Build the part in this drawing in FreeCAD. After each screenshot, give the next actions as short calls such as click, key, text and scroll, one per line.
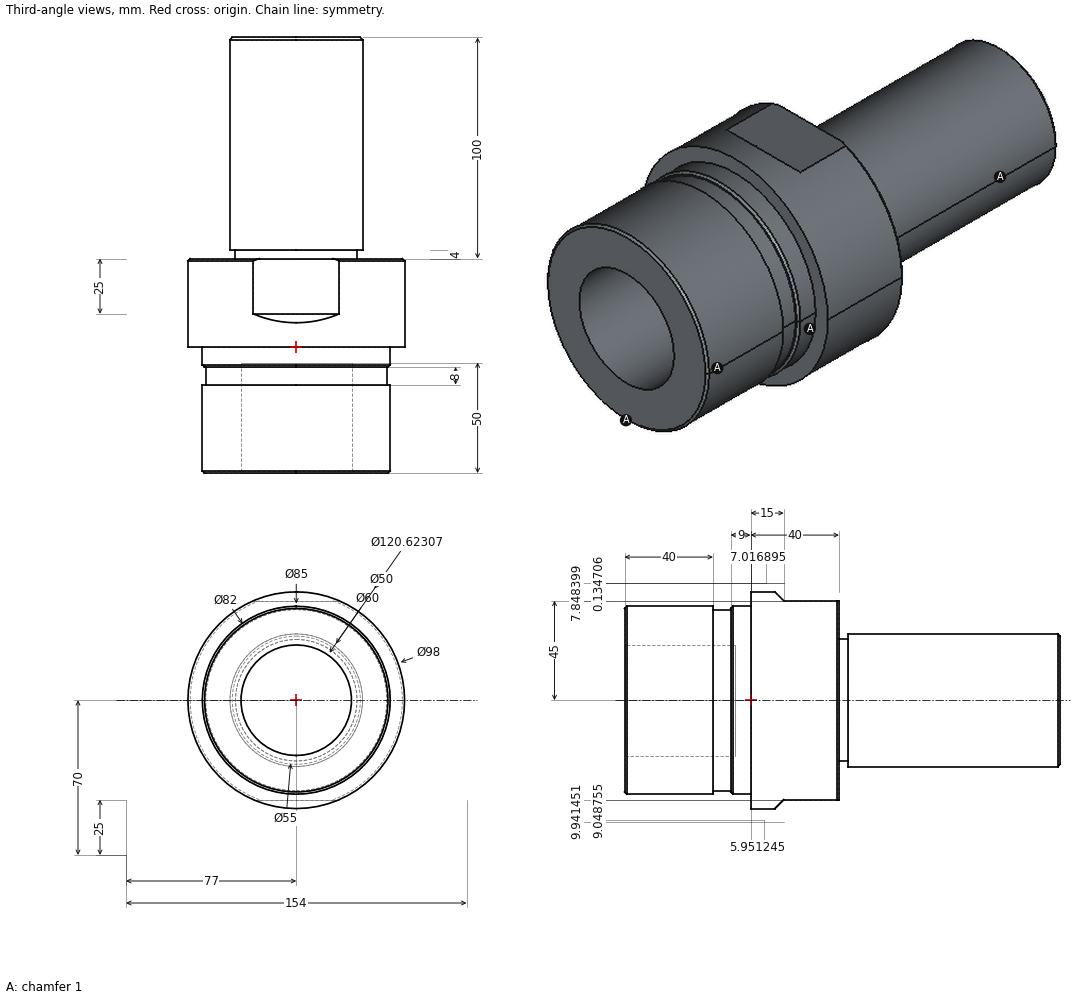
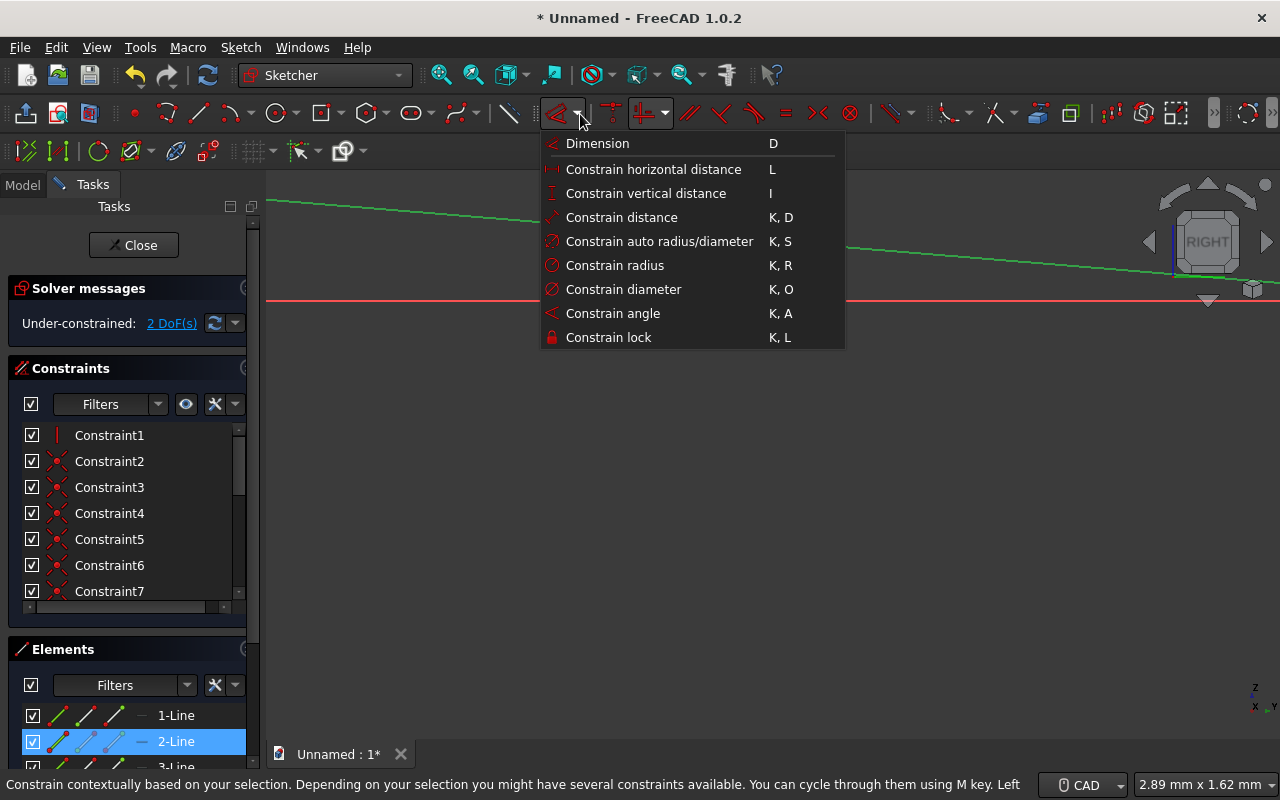
click(693, 193)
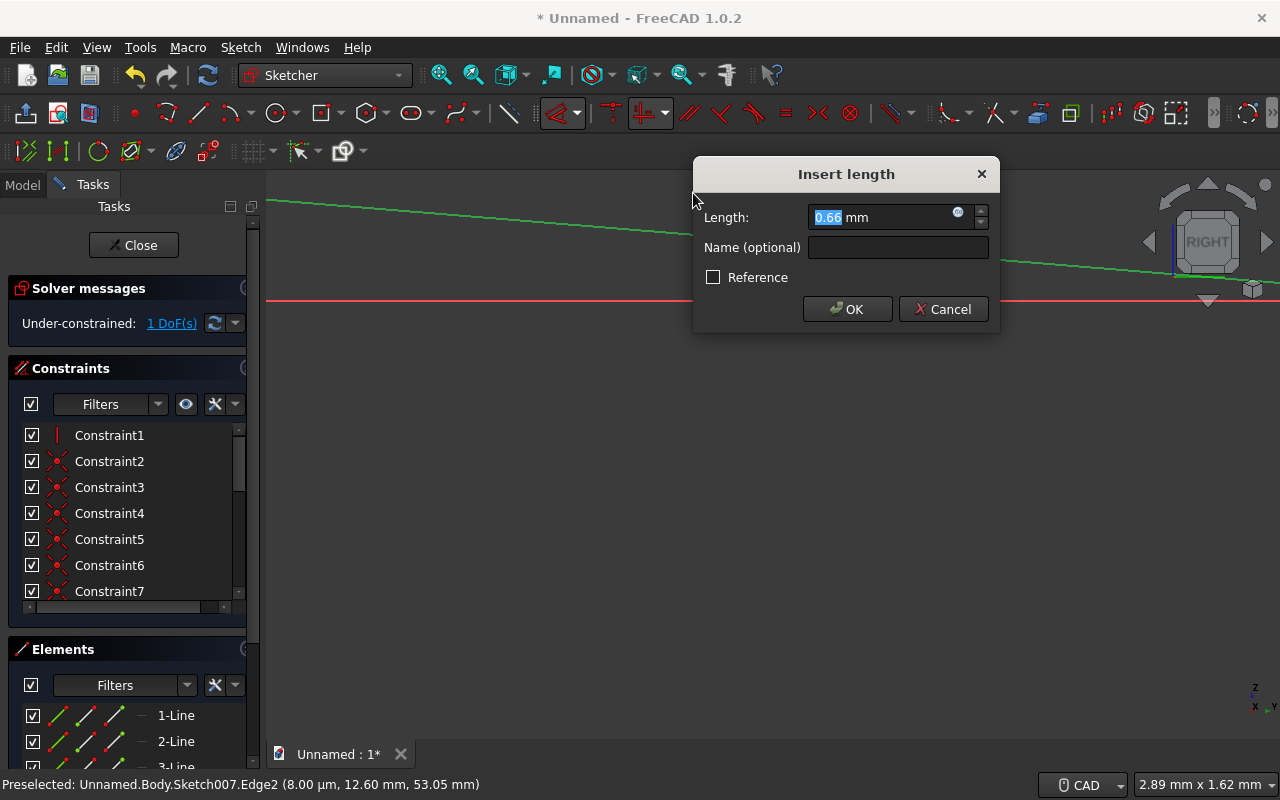
text(0.134706)
key(Return)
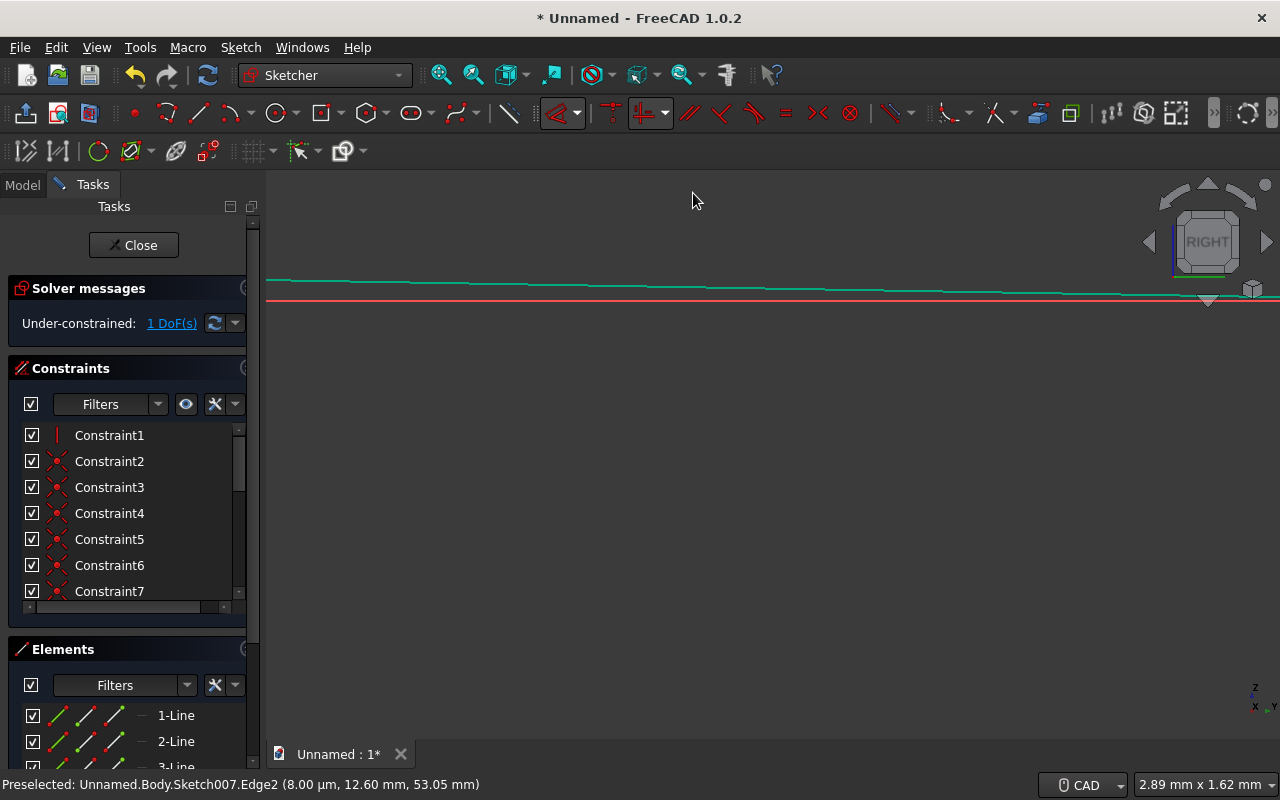
scroll(704, 454, down, 15)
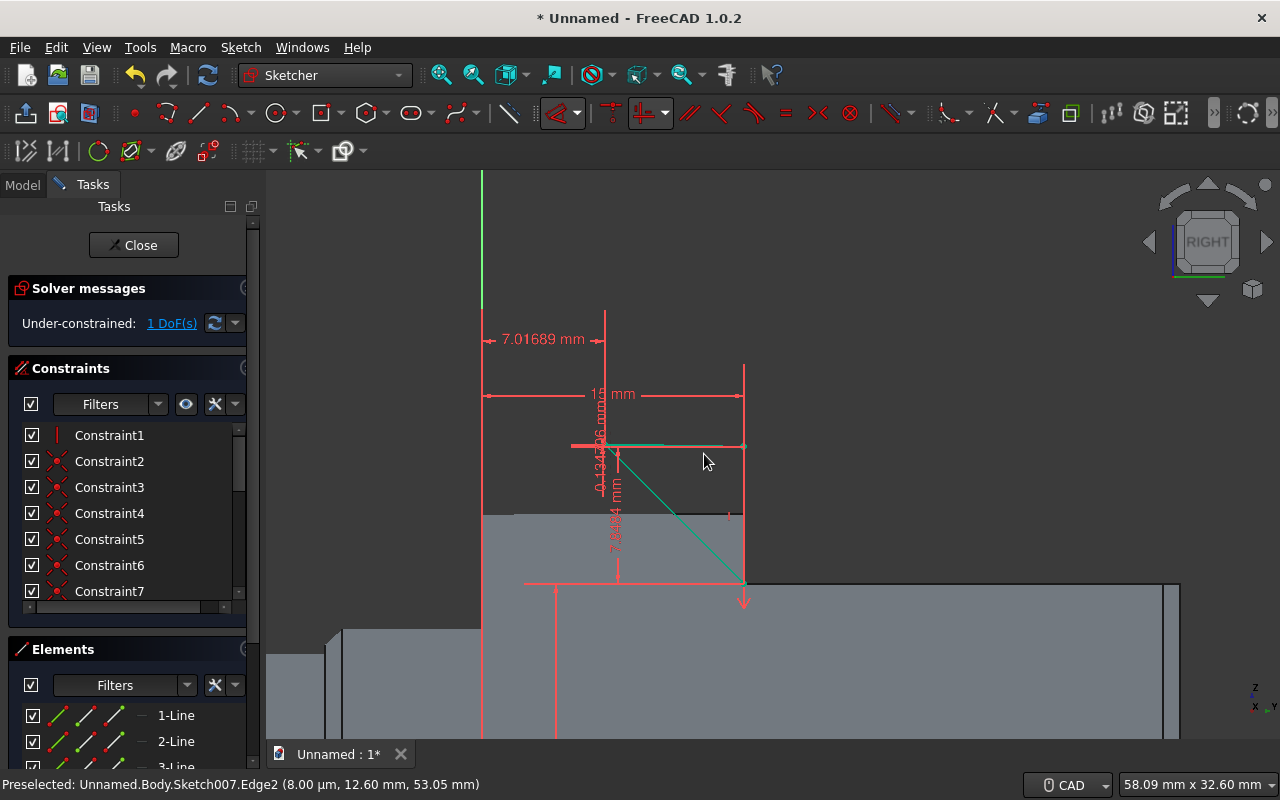
scroll(728, 219, down, 8)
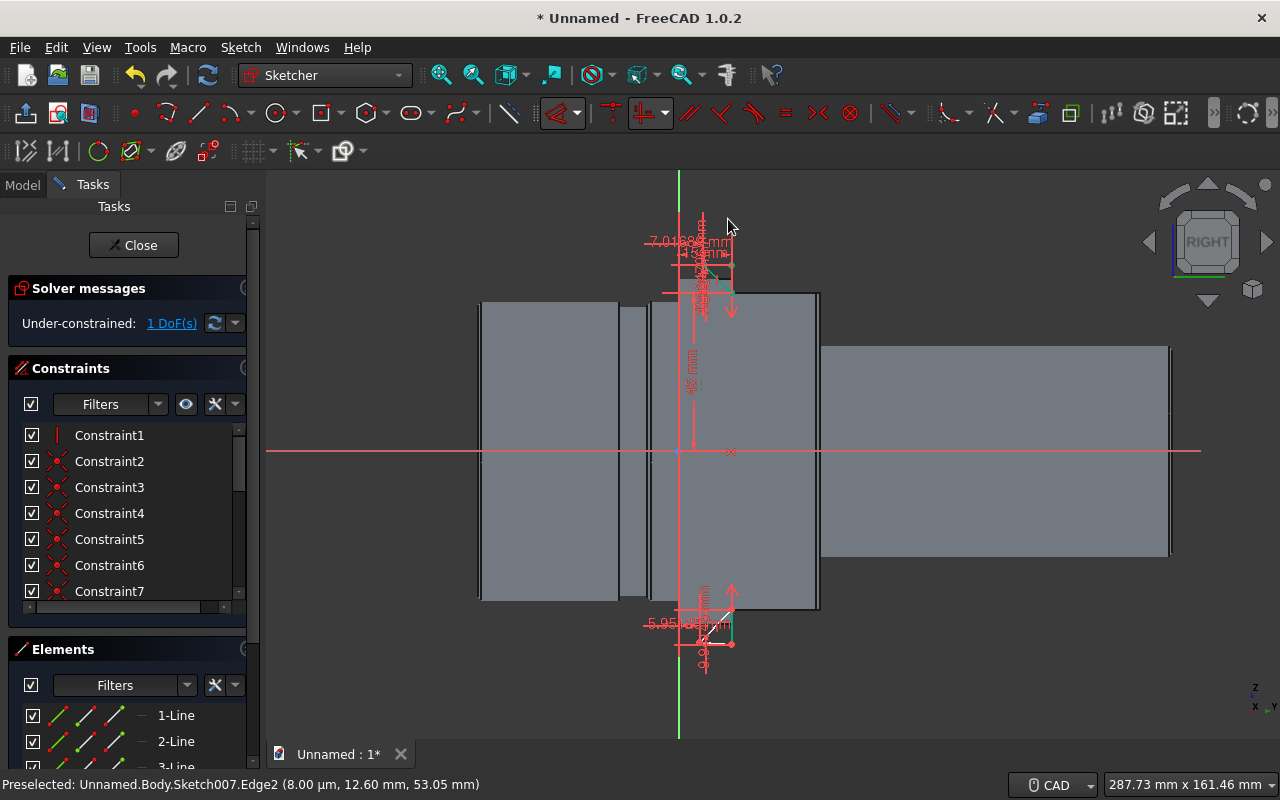
scroll(722, 620, up, 2)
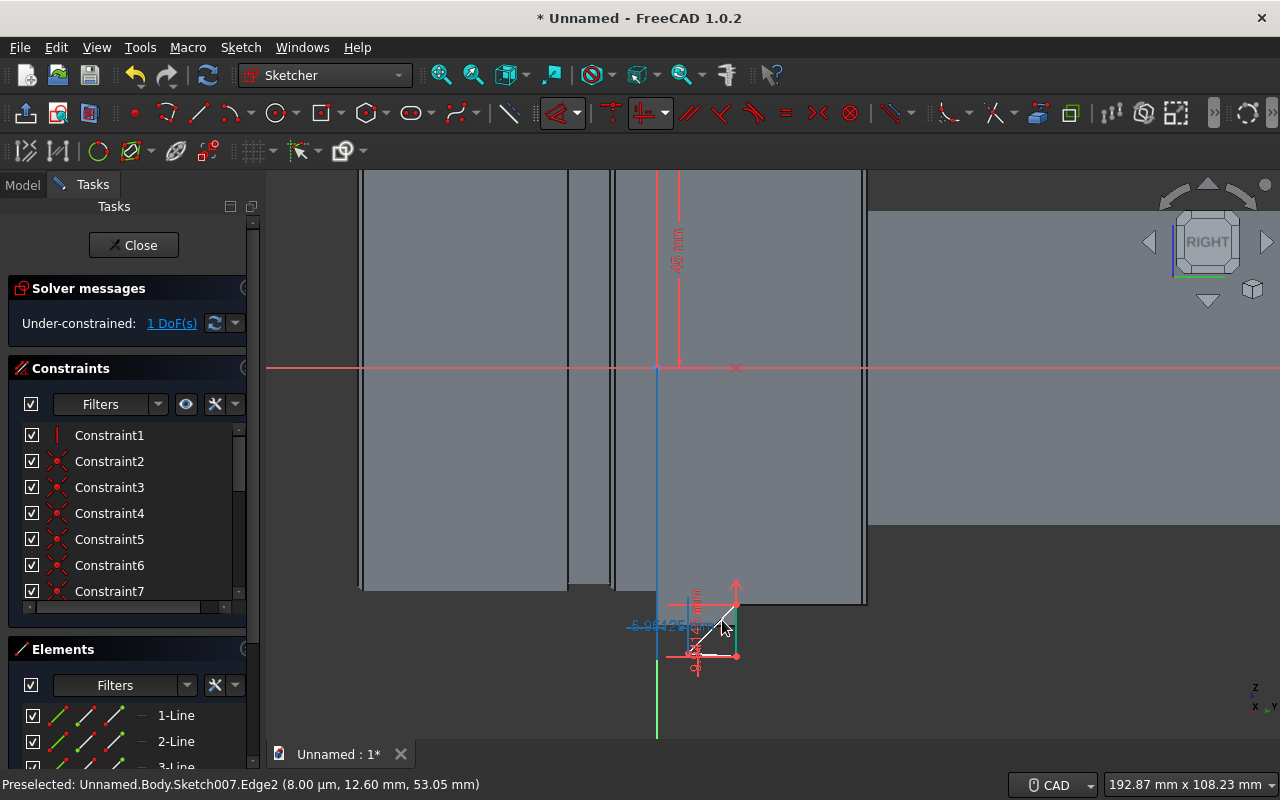
click(722, 619)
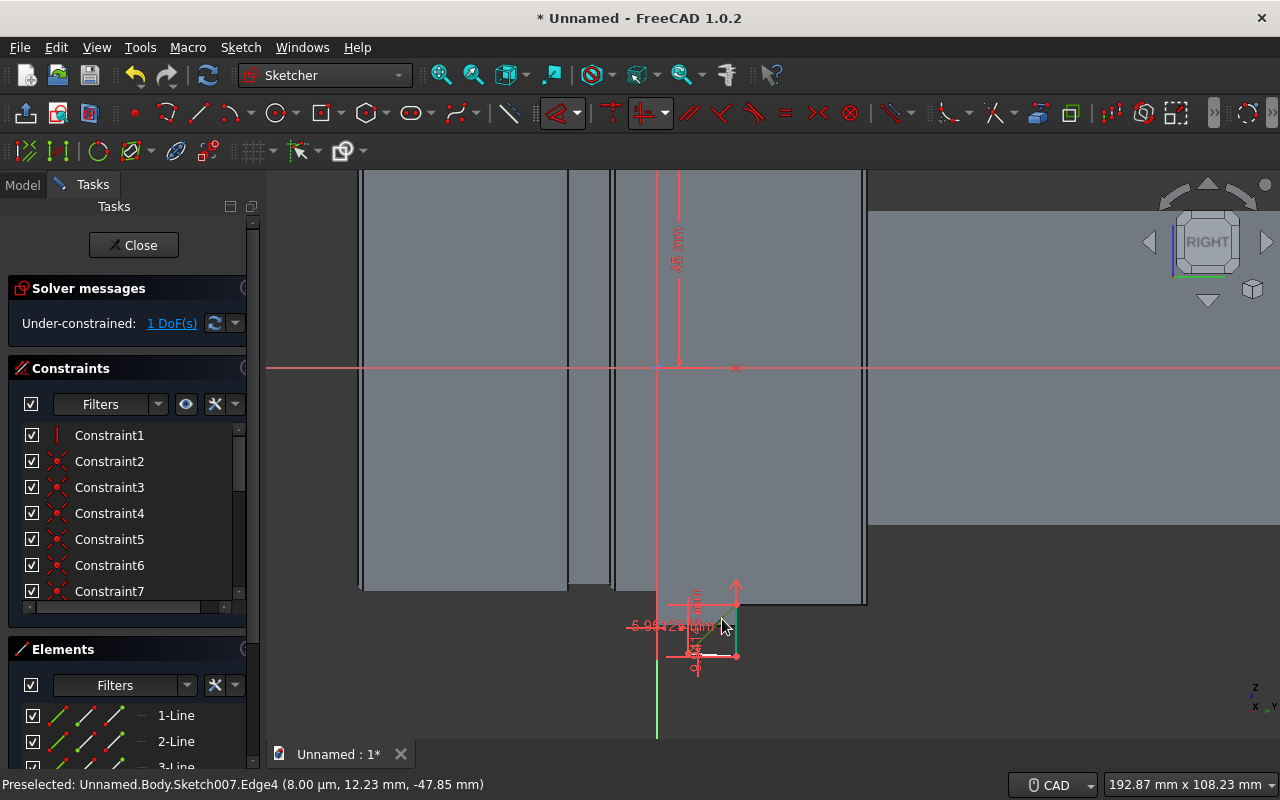
key(i)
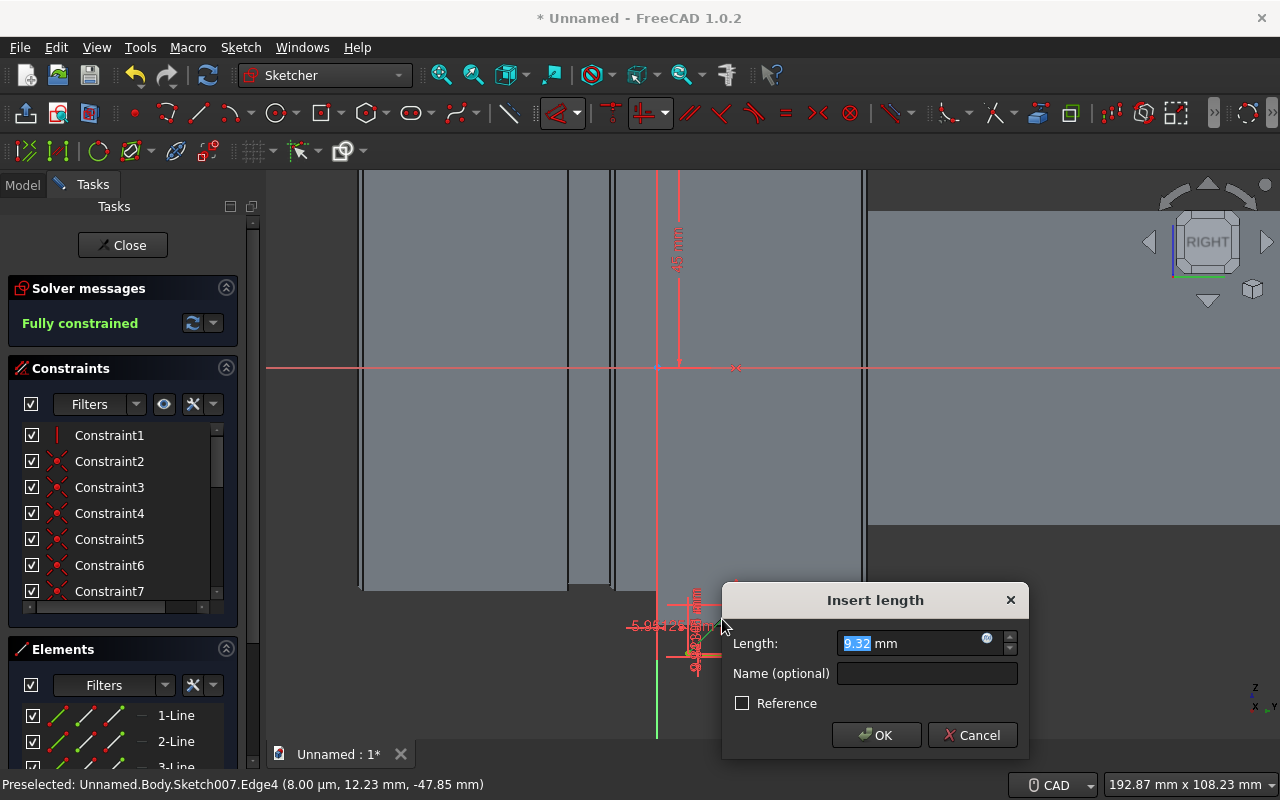
text(9.048755)
key(Return)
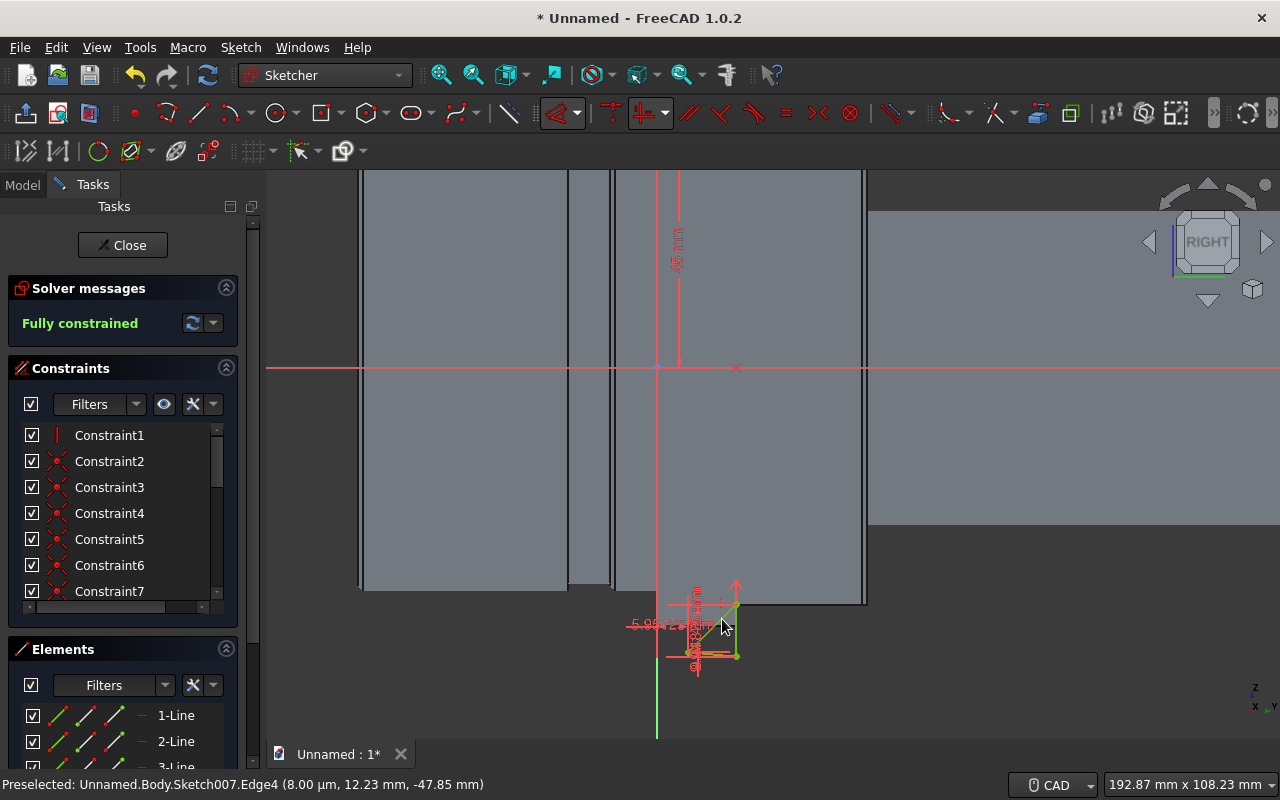
click(123, 245)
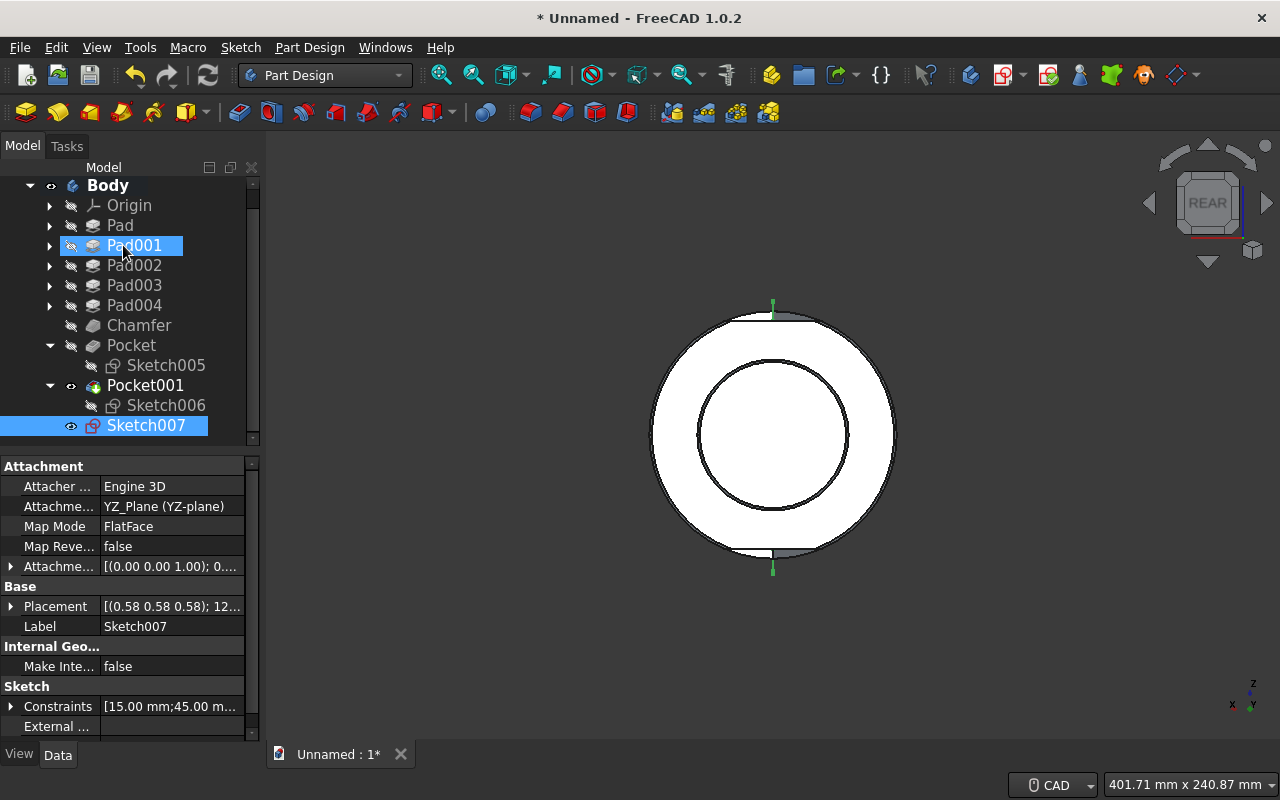
click(240, 112)